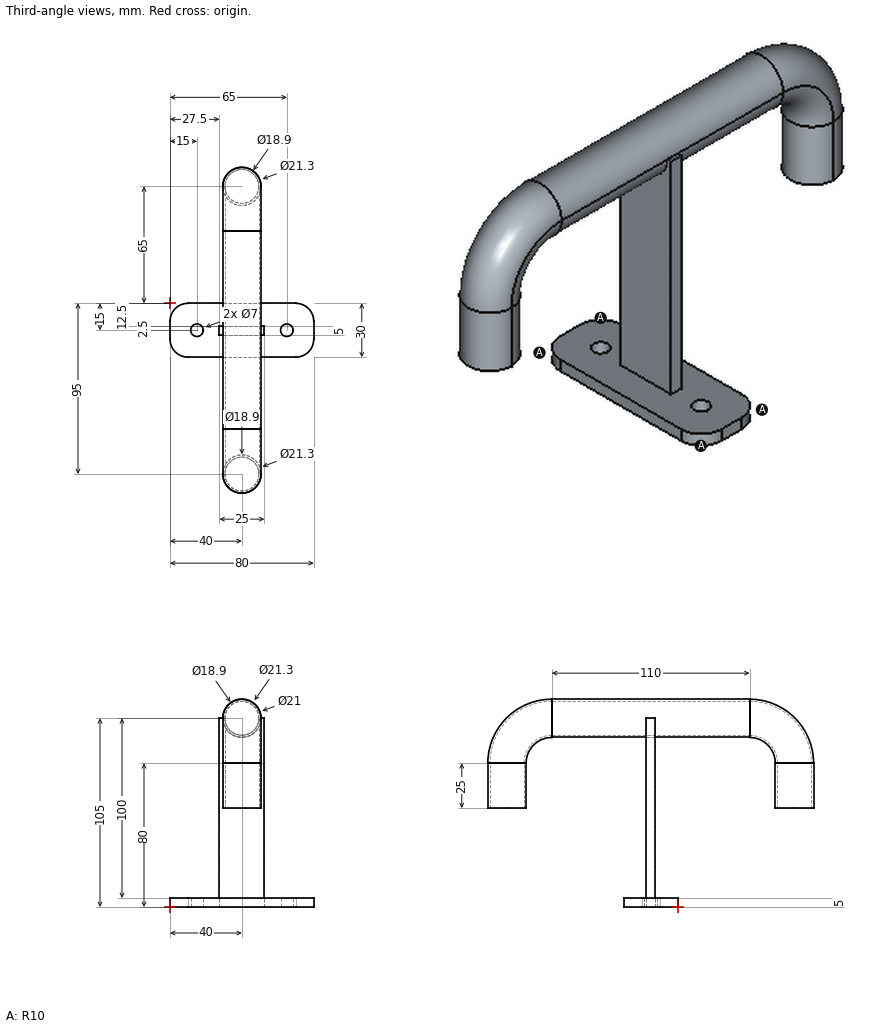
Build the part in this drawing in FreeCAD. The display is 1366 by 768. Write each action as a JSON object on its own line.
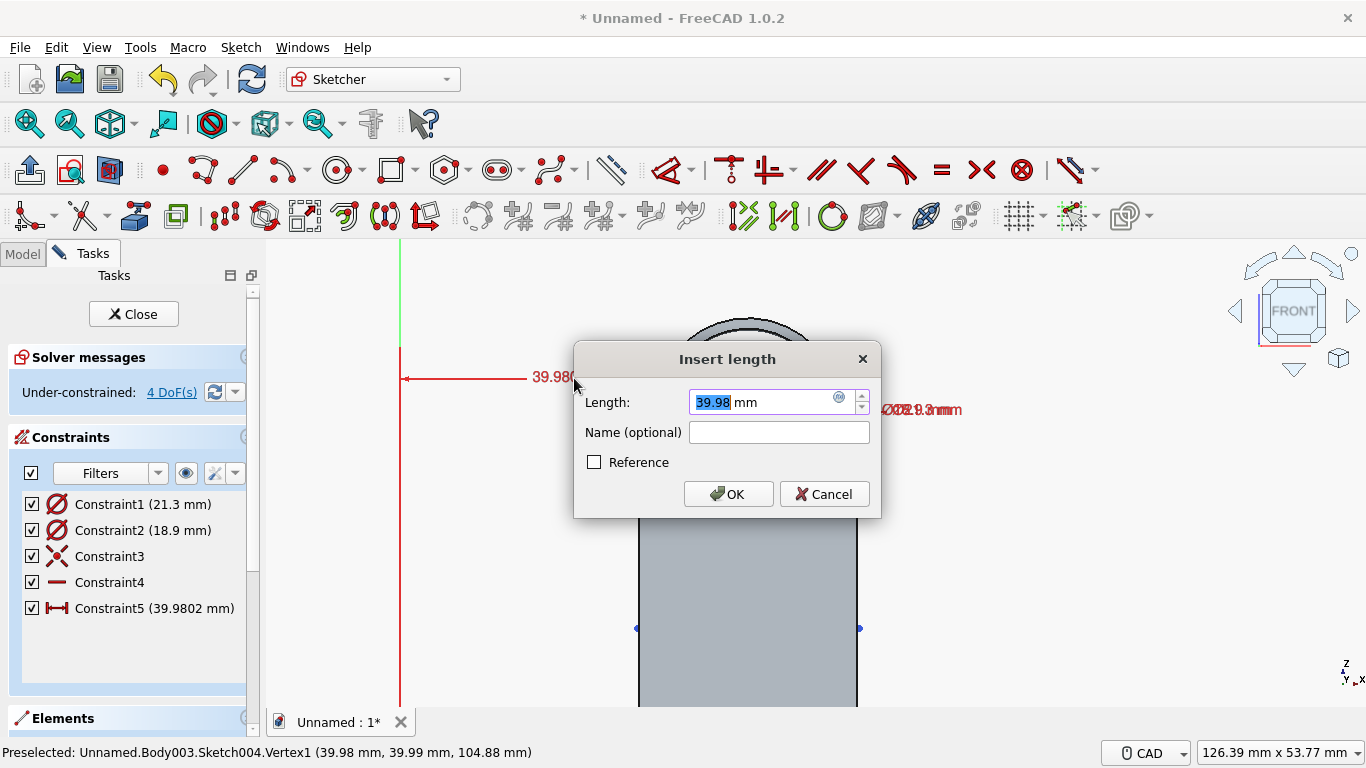
{"action": "type", "text": "40"}
{"action": "key", "text": "Return"}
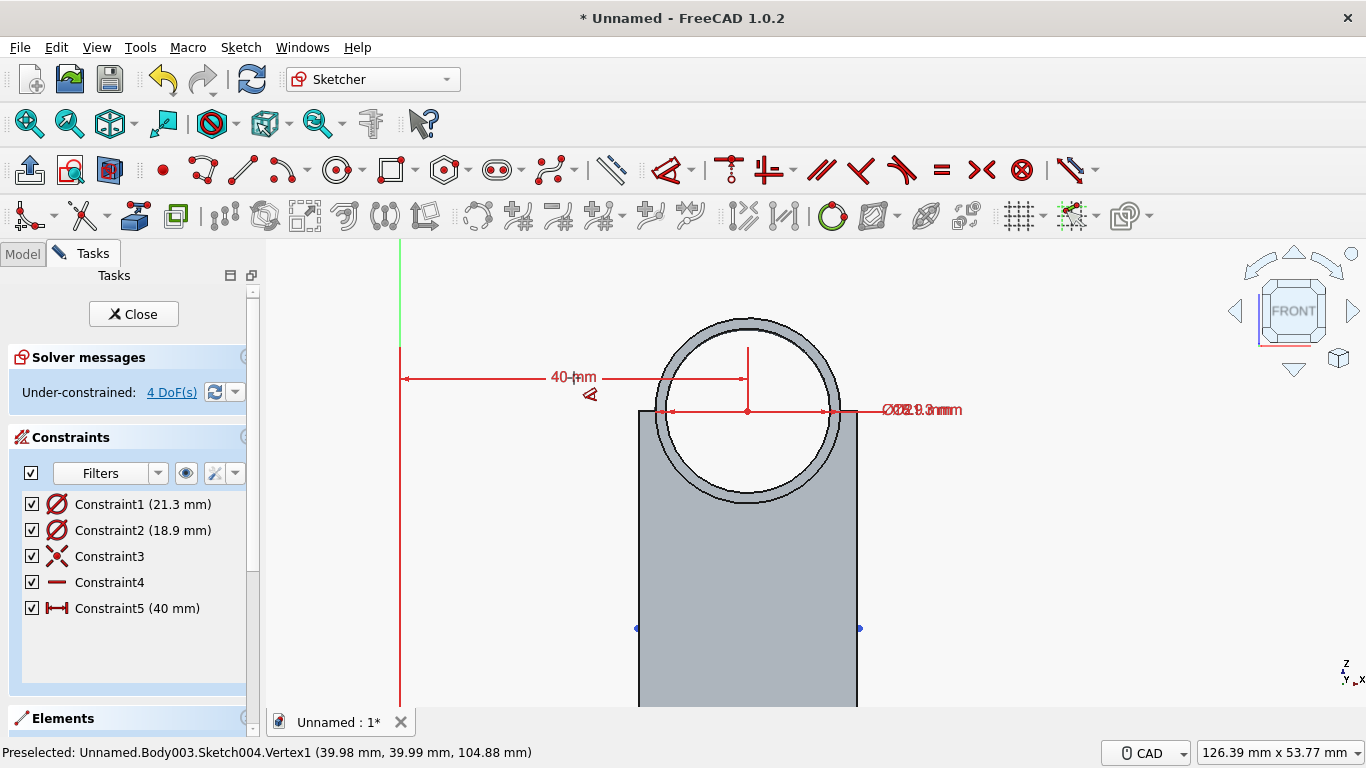
{"action": "left_click", "coordinate": [859, 629]}
{"action": "left_click", "coordinate": [366, 654]}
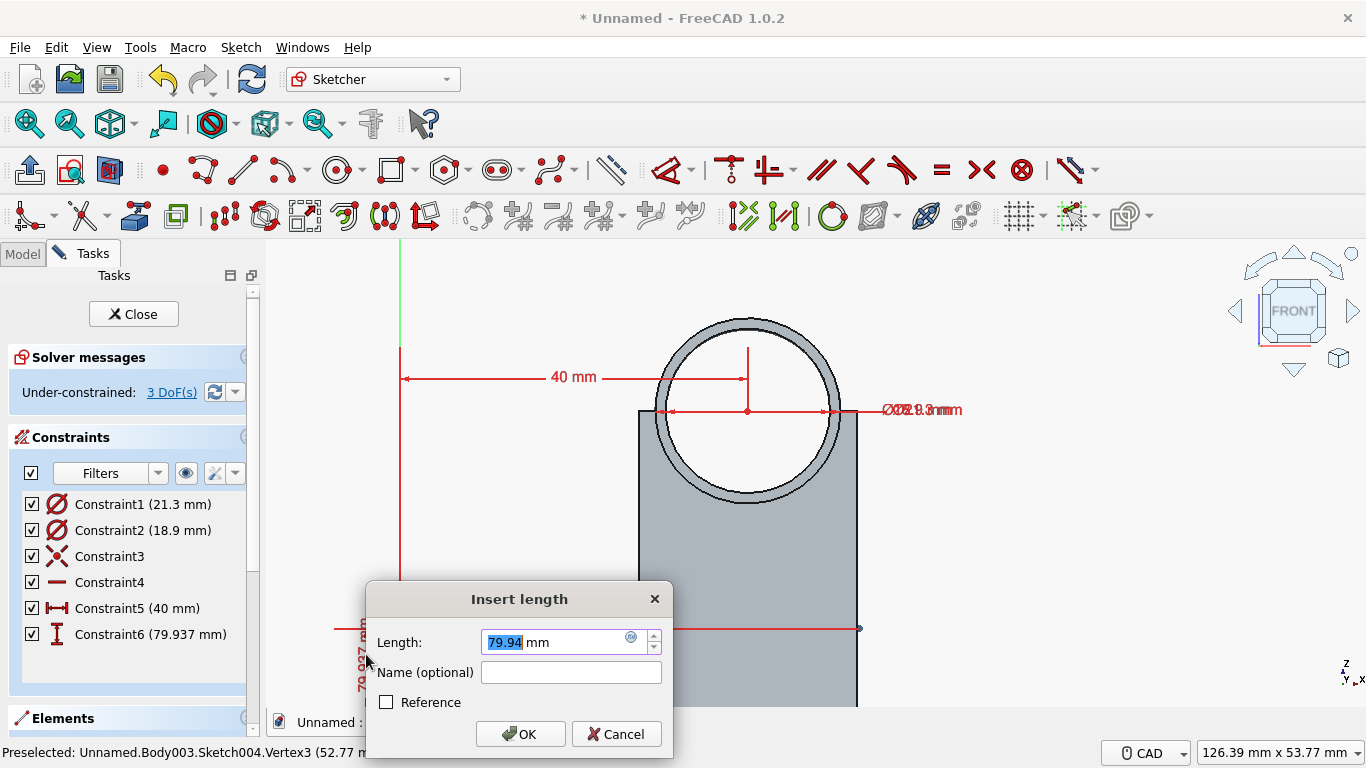
{"action": "type", "text": "80"}
{"action": "key", "text": "Return"}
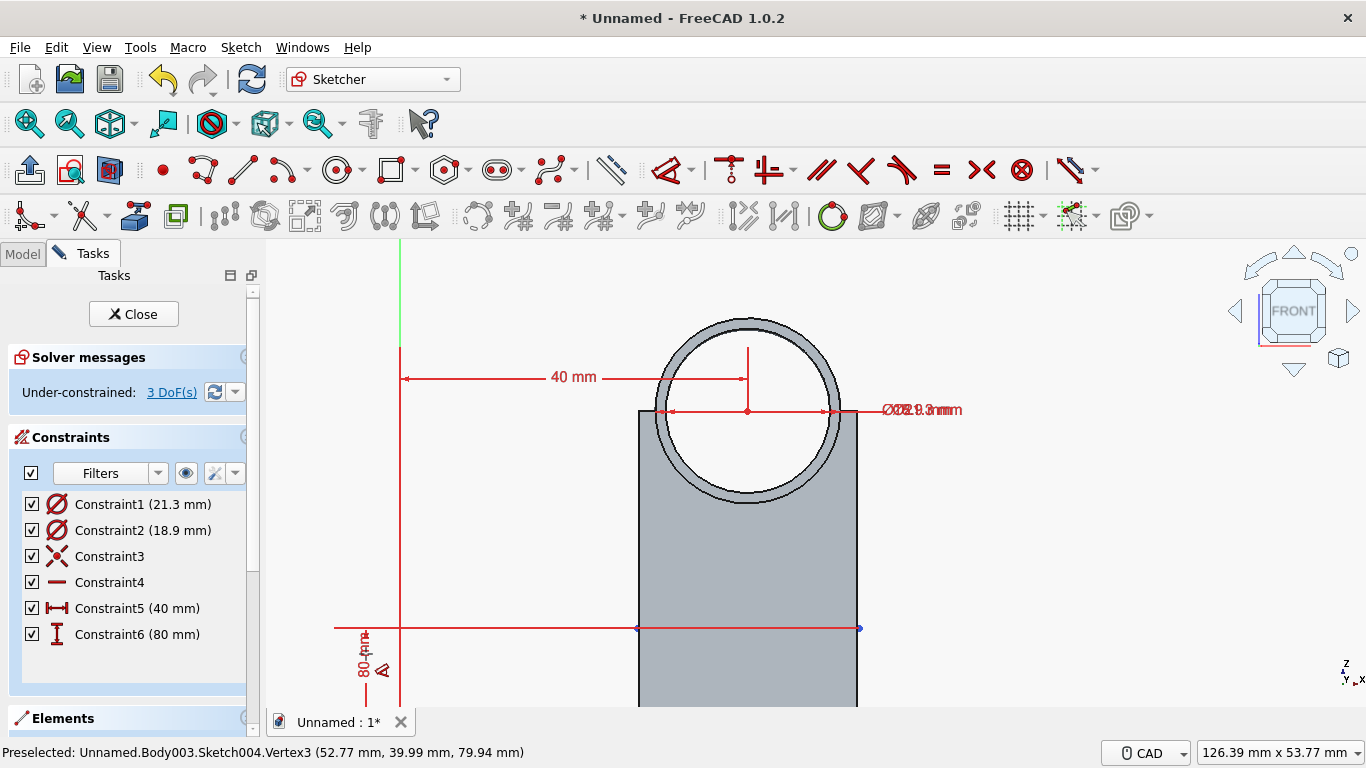
{"action": "left_click", "coordinate": [748, 412]}
{"action": "left_click", "coordinate": [366, 545]}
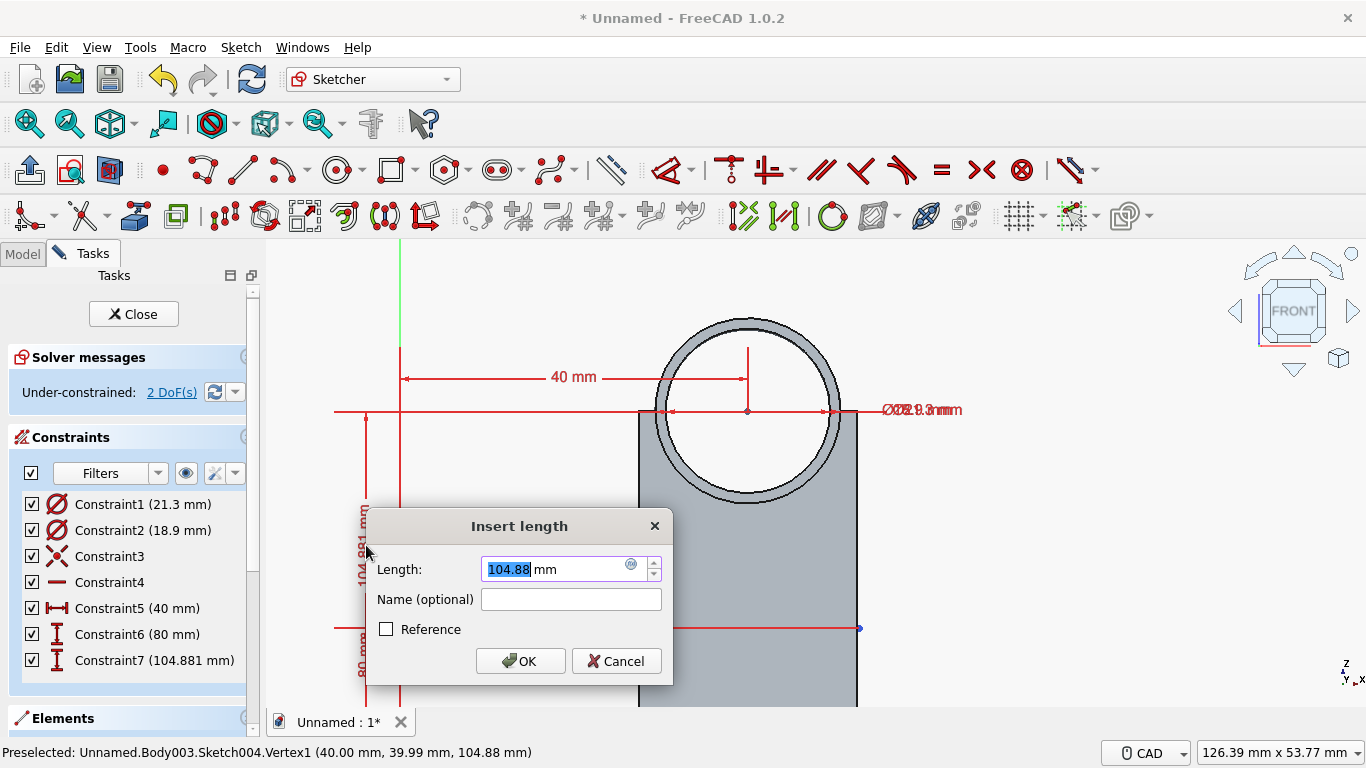
{"action": "type", "text": "105"}
{"action": "key", "text": "Return"}
{"action": "key", "text": "Escape"}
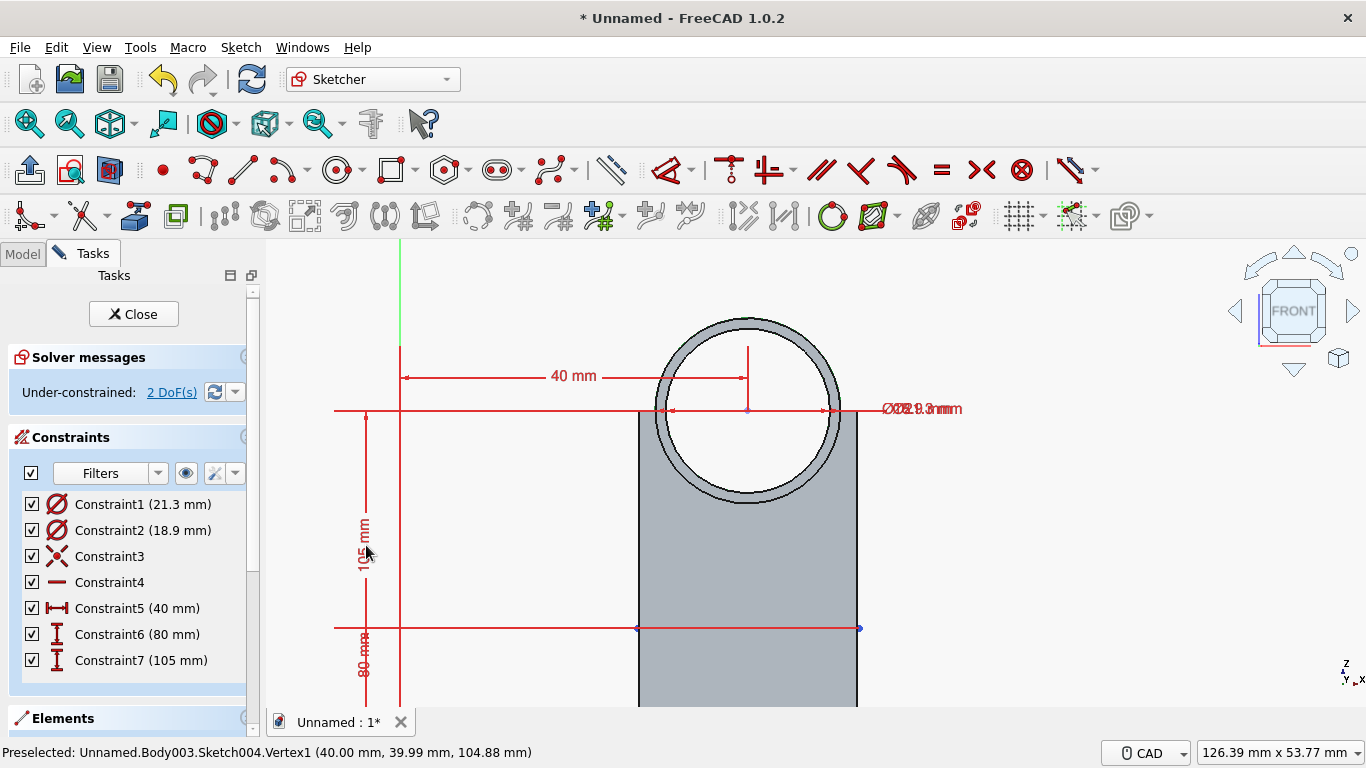
{"action": "left_click", "coordinate": [134, 314]}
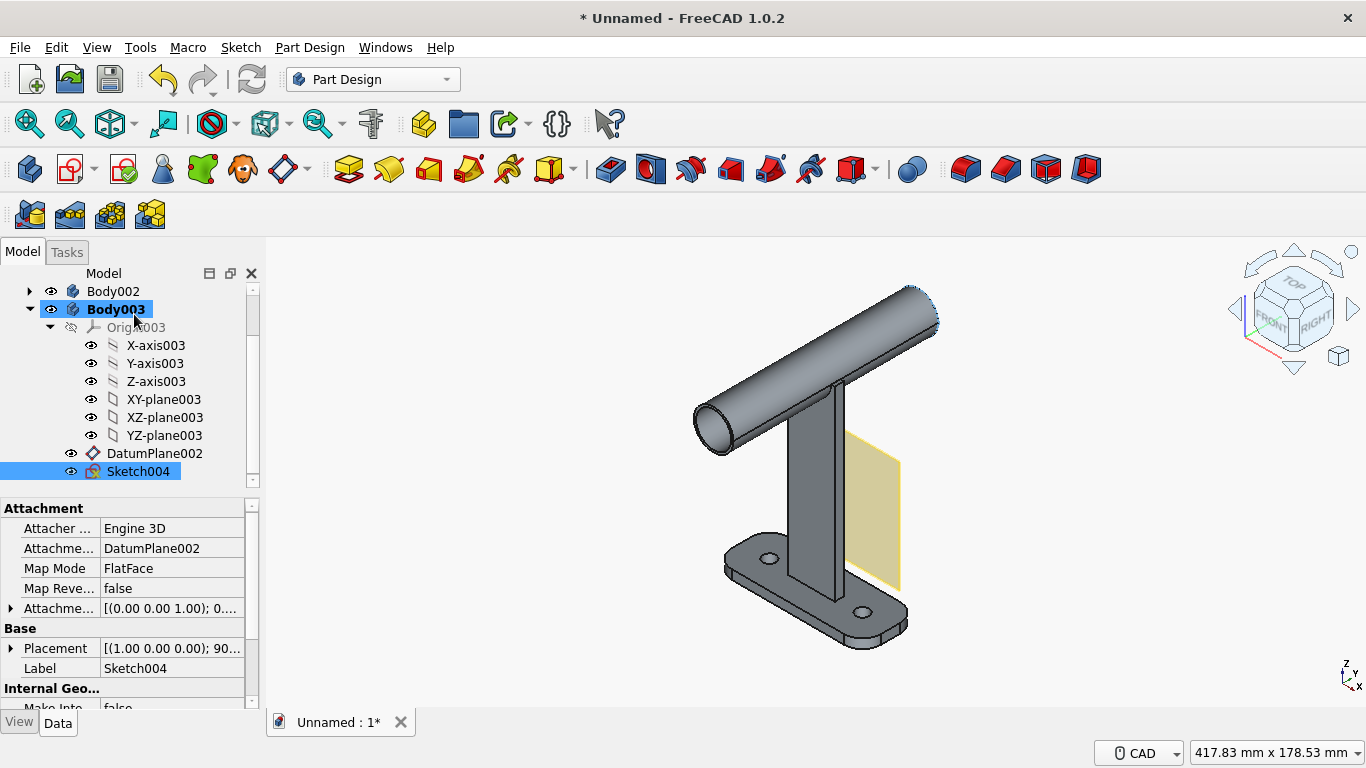
{"action": "left_click", "coordinate": [390, 170]}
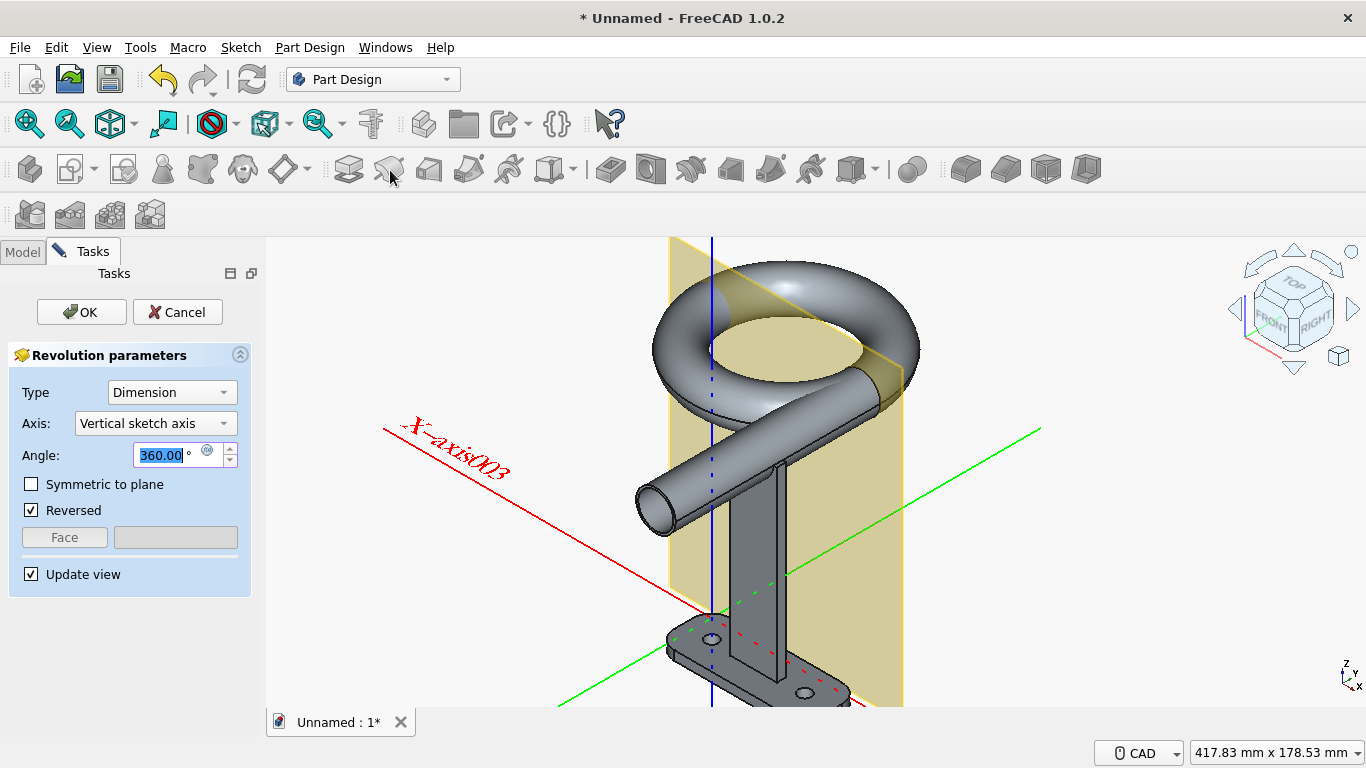
{"action": "left_click", "coordinate": [156, 424]}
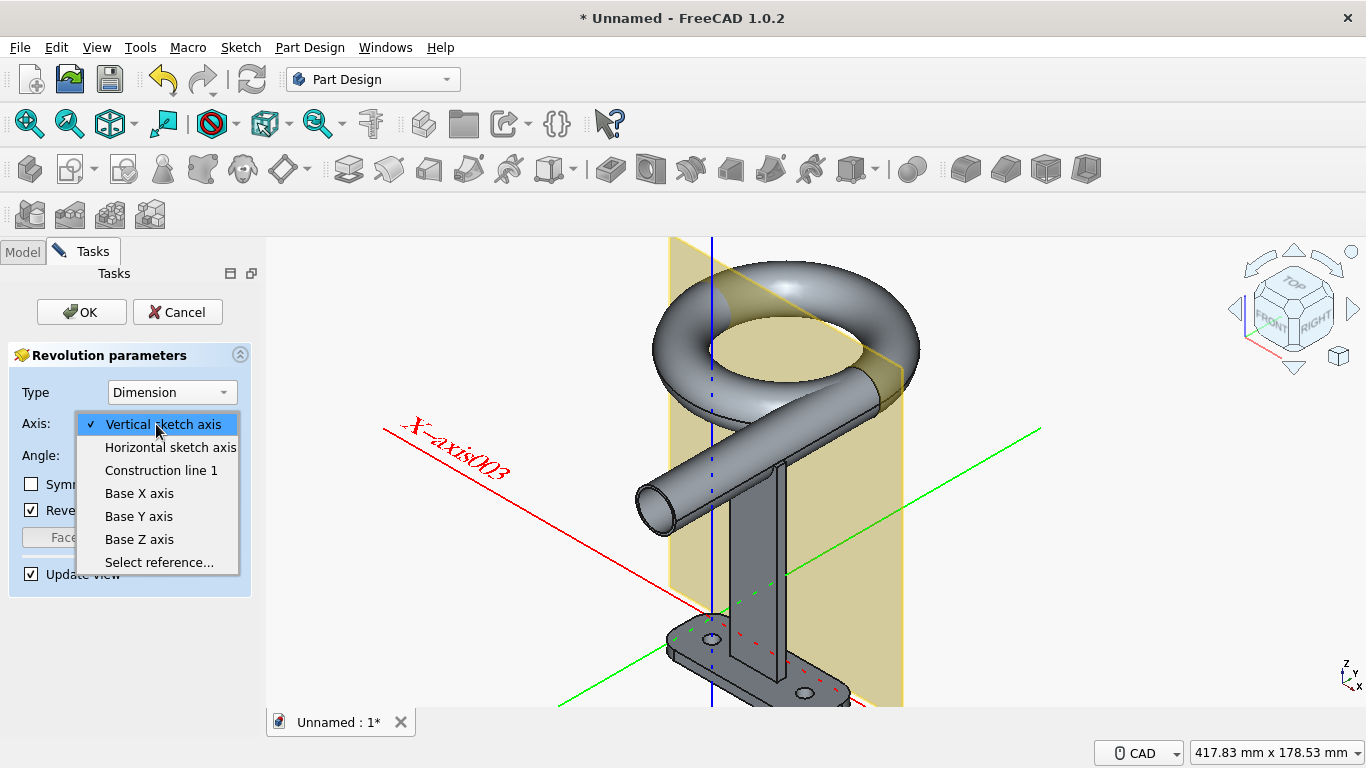
{"action": "left_click", "coordinate": [156, 470]}